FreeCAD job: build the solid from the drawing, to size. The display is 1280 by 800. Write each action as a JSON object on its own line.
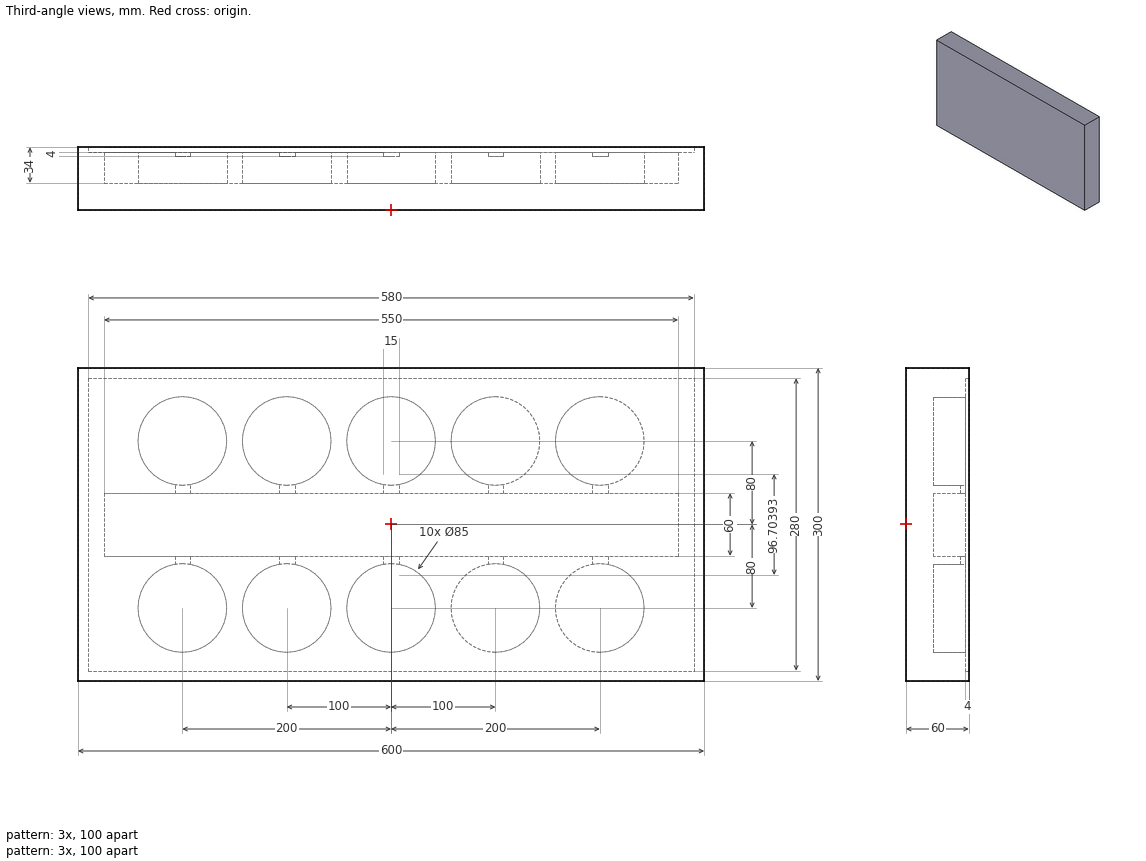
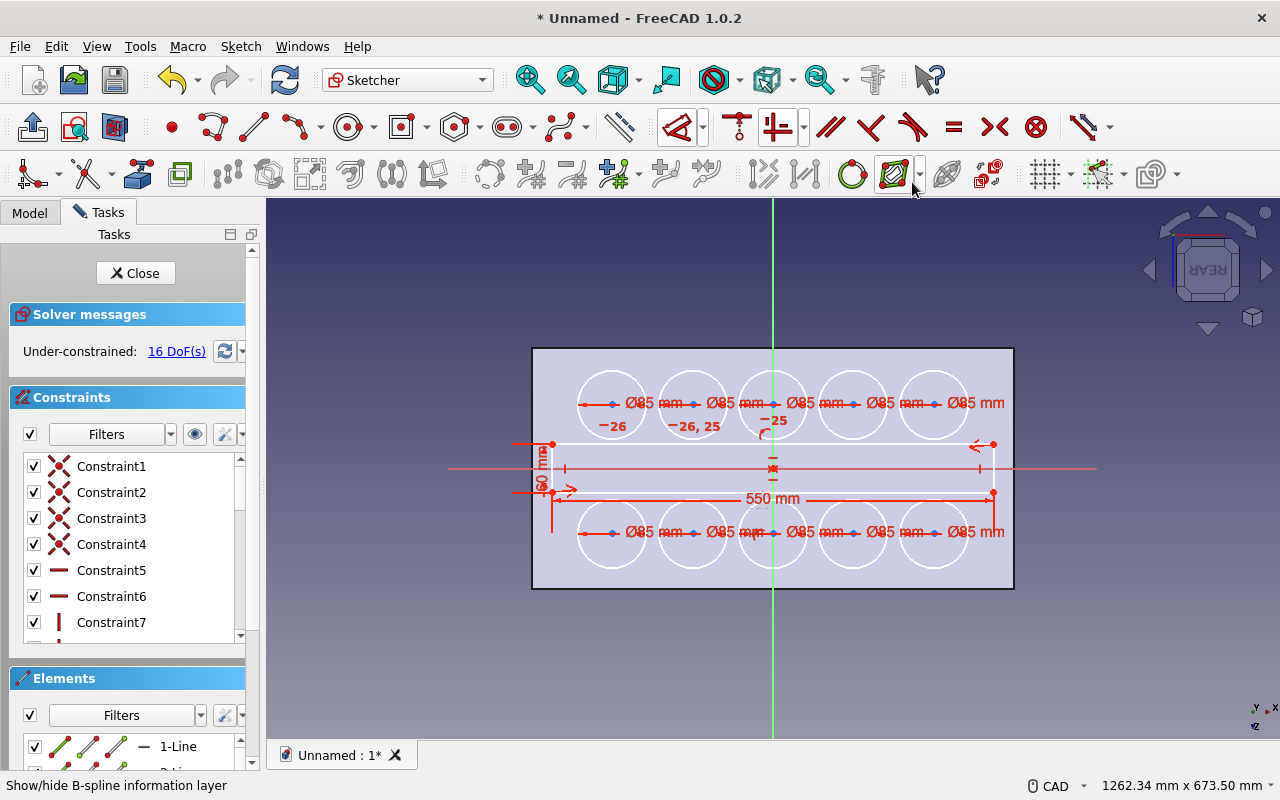
{"action": "left_click", "coordinate": [773, 405]}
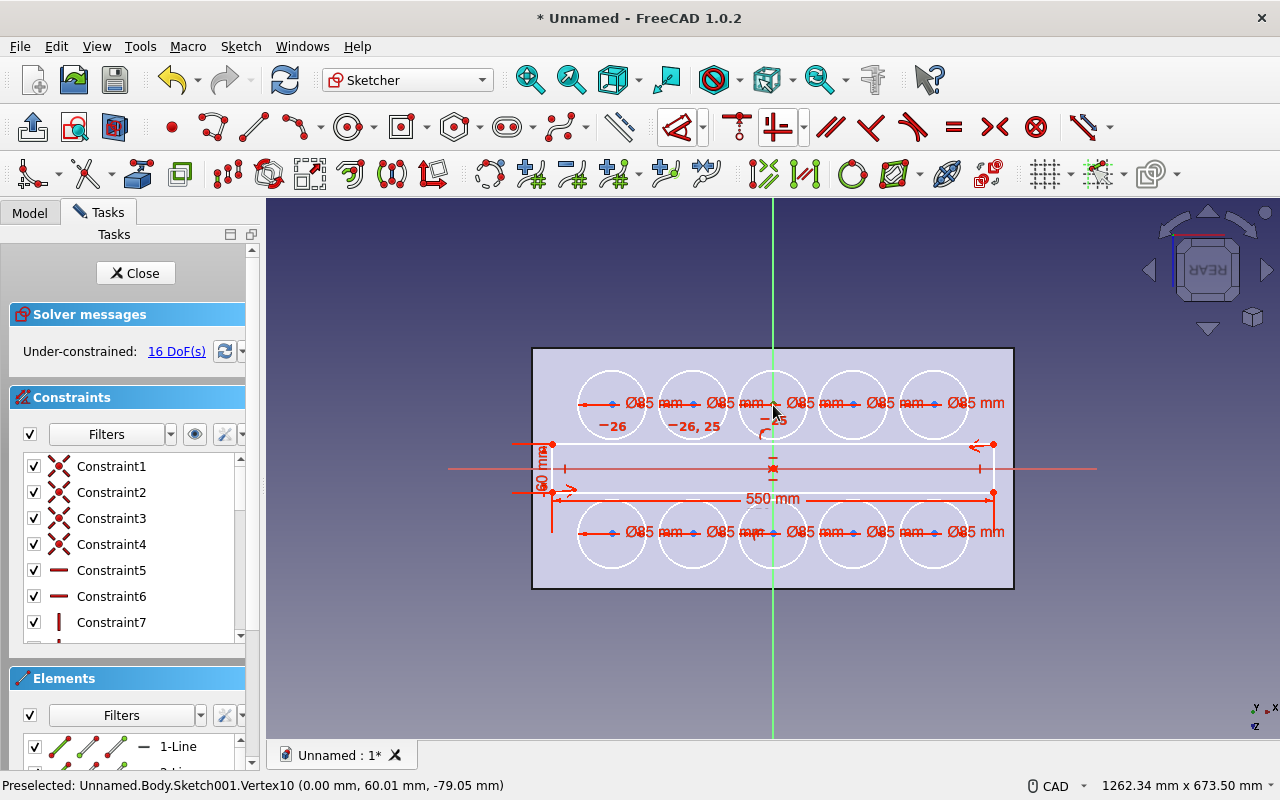
{"action": "left_click", "coordinate": [934, 405]}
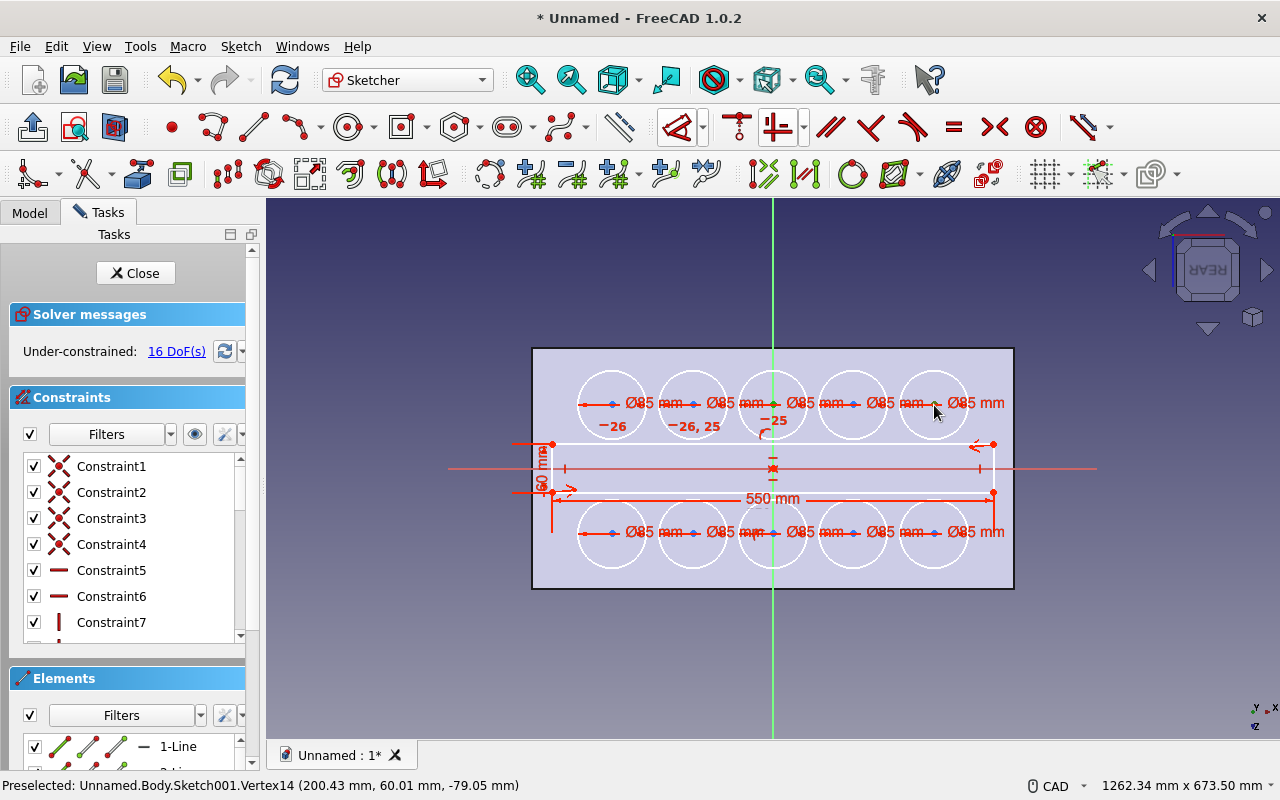
{"action": "left_click", "coordinate": [804, 128]}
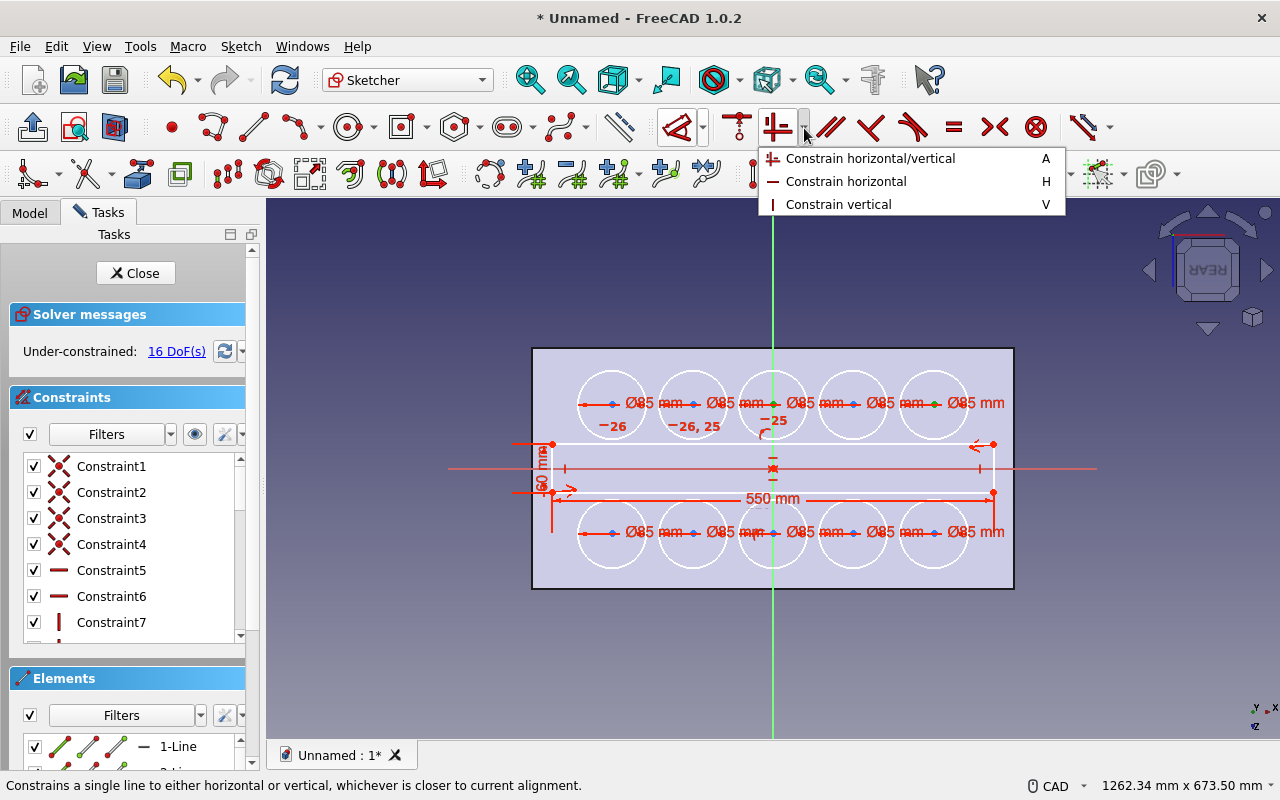
{"action": "left_click", "coordinate": [912, 182]}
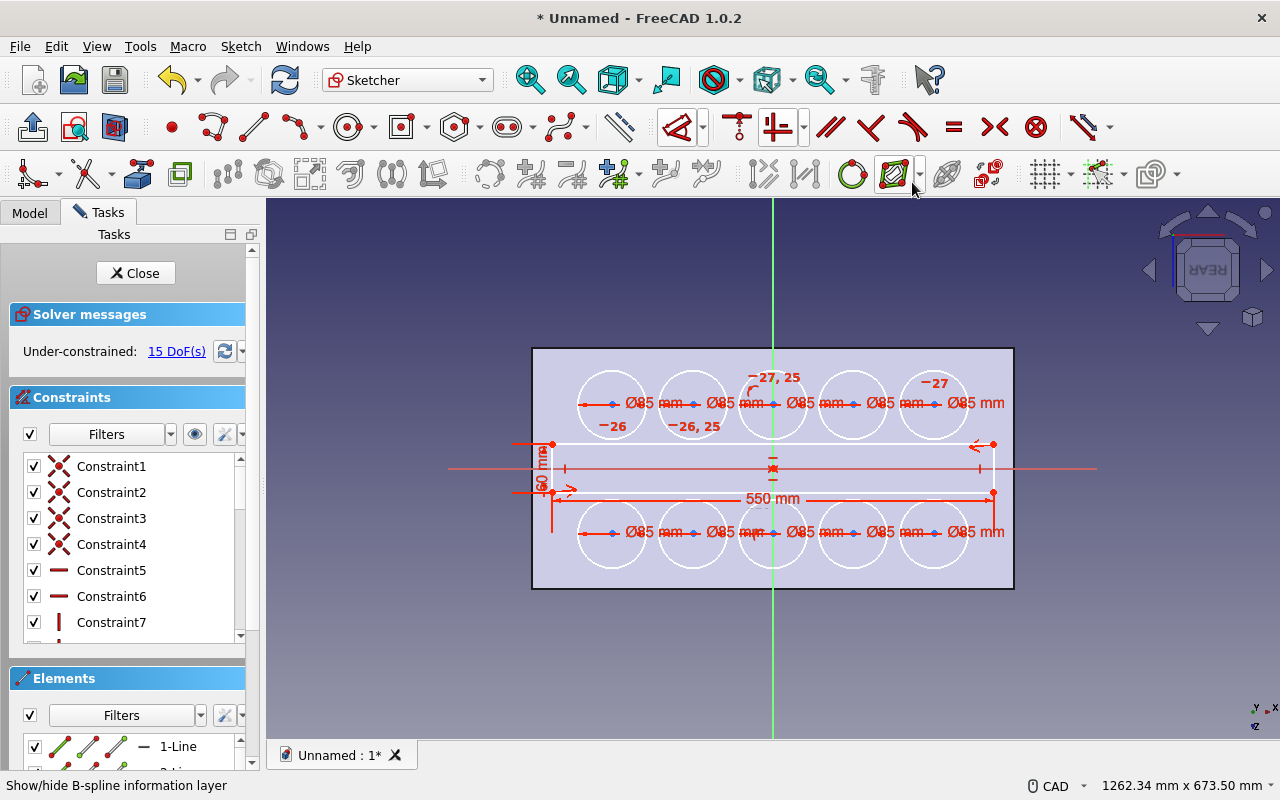
{"action": "left_click", "coordinate": [773, 405]}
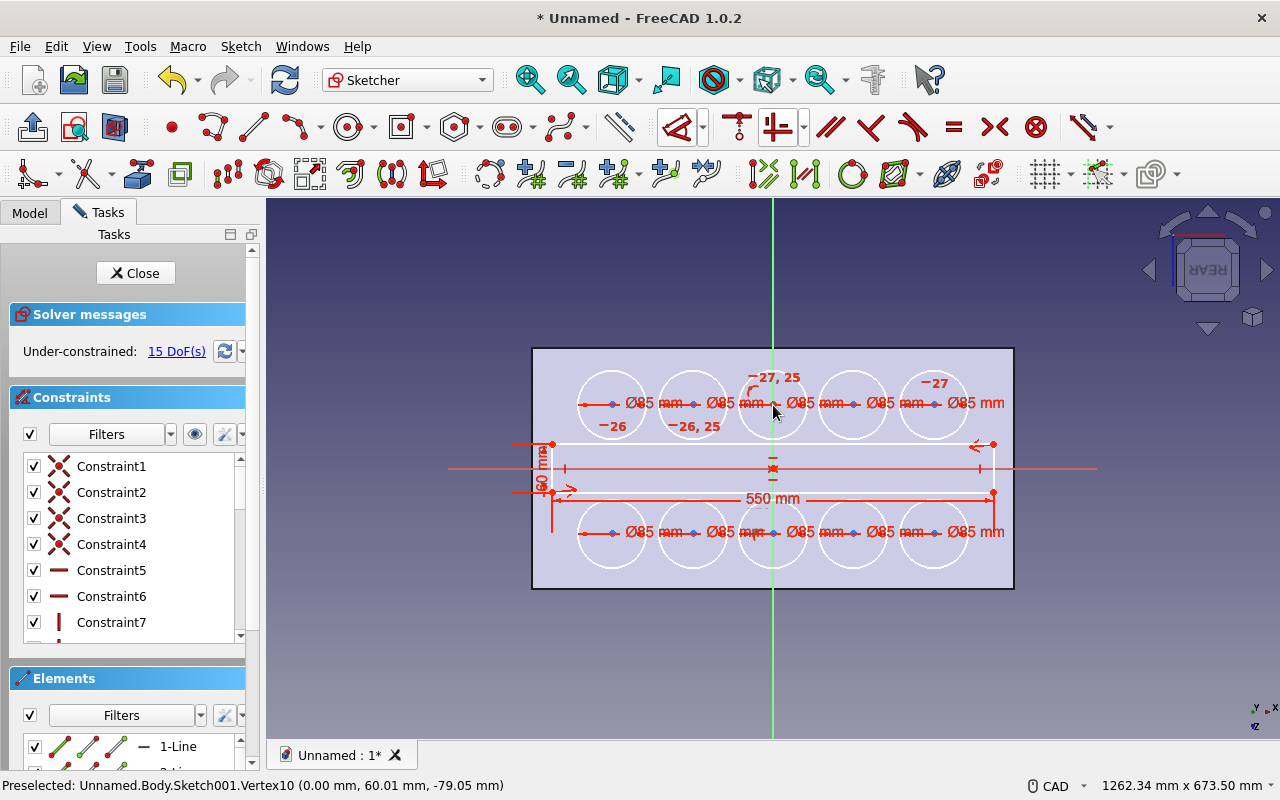
{"action": "left_click", "coordinate": [853, 405]}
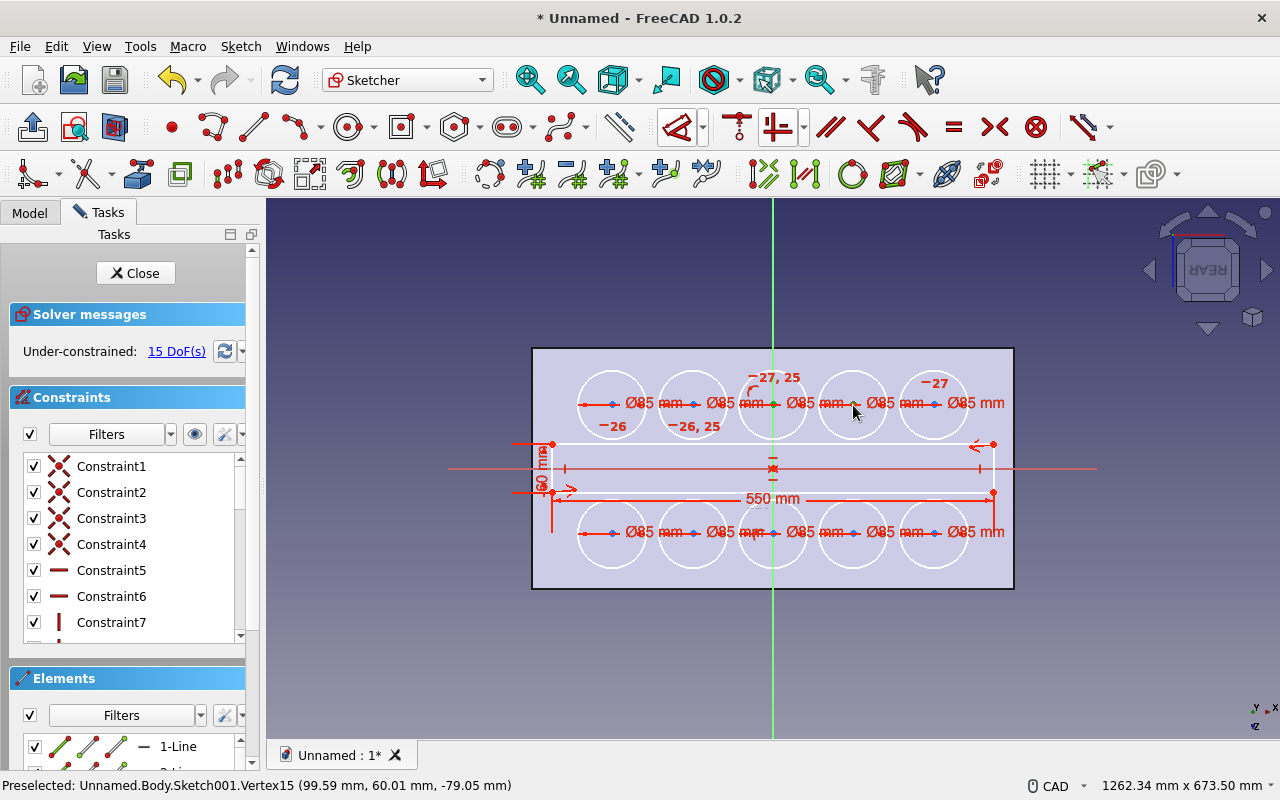
{"action": "left_click", "coordinate": [804, 128]}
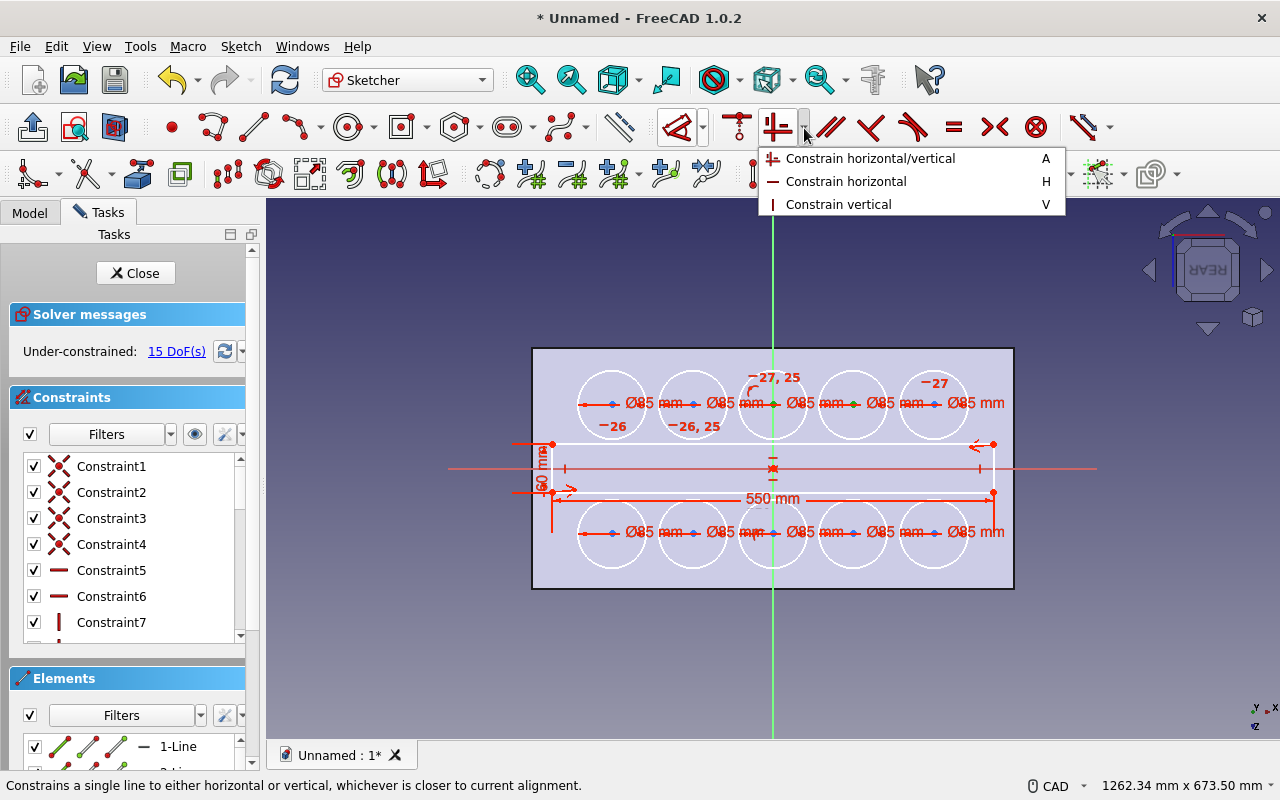
{"action": "left_click", "coordinate": [912, 182]}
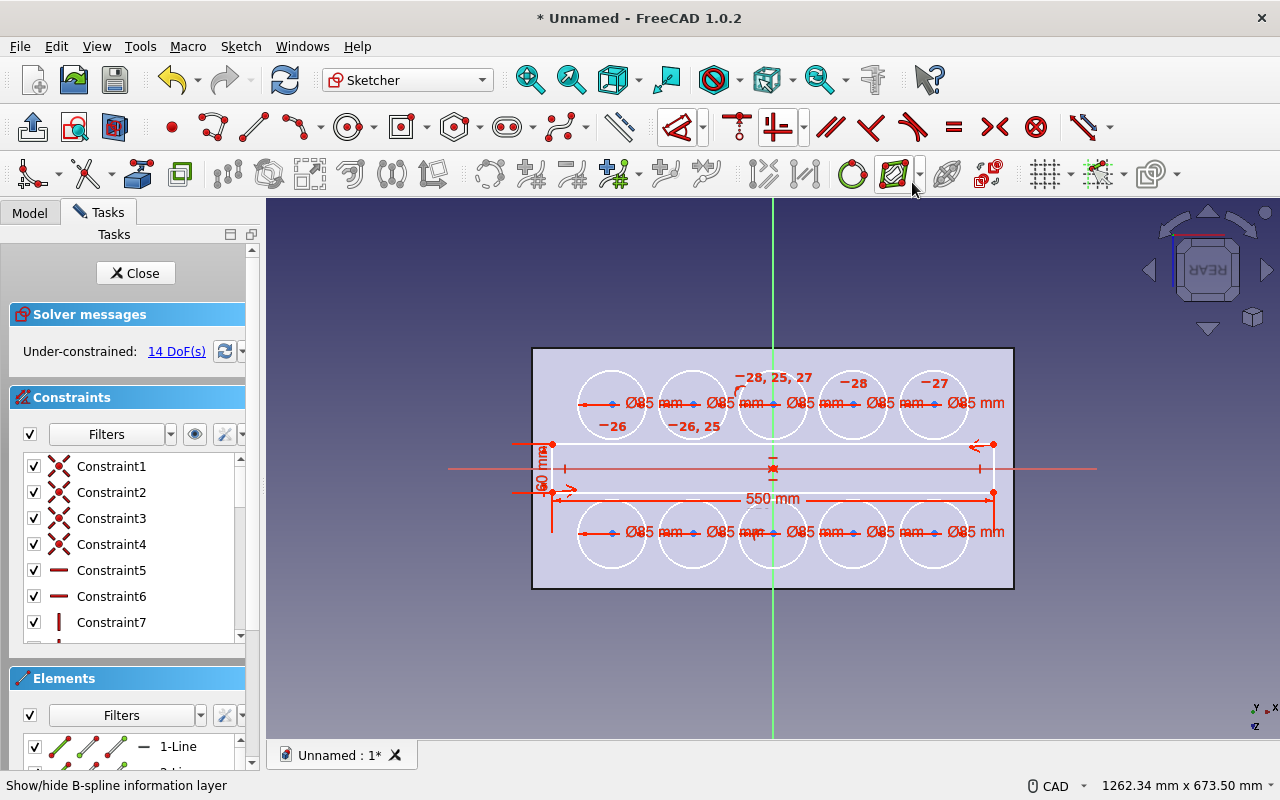
{"action": "left_click", "coordinate": [934, 405]}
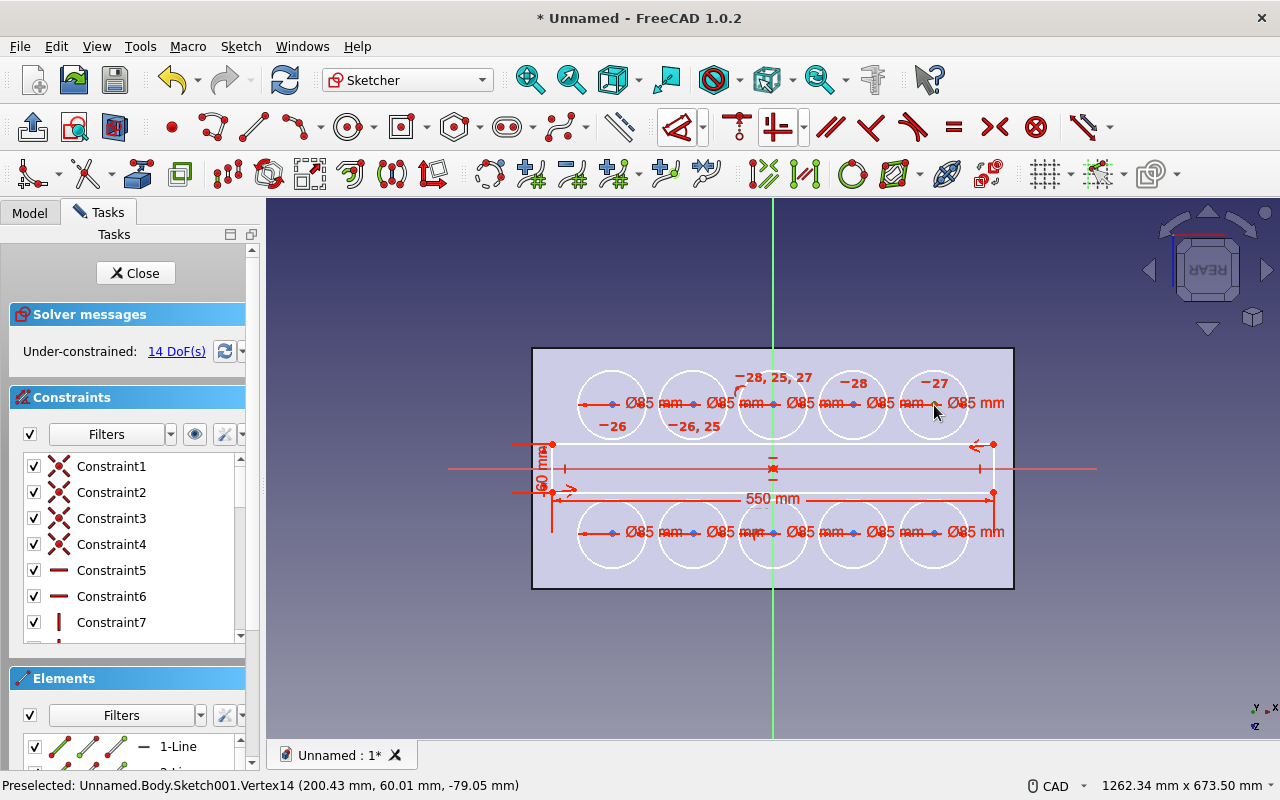
{"action": "left_click", "coordinate": [934, 534]}